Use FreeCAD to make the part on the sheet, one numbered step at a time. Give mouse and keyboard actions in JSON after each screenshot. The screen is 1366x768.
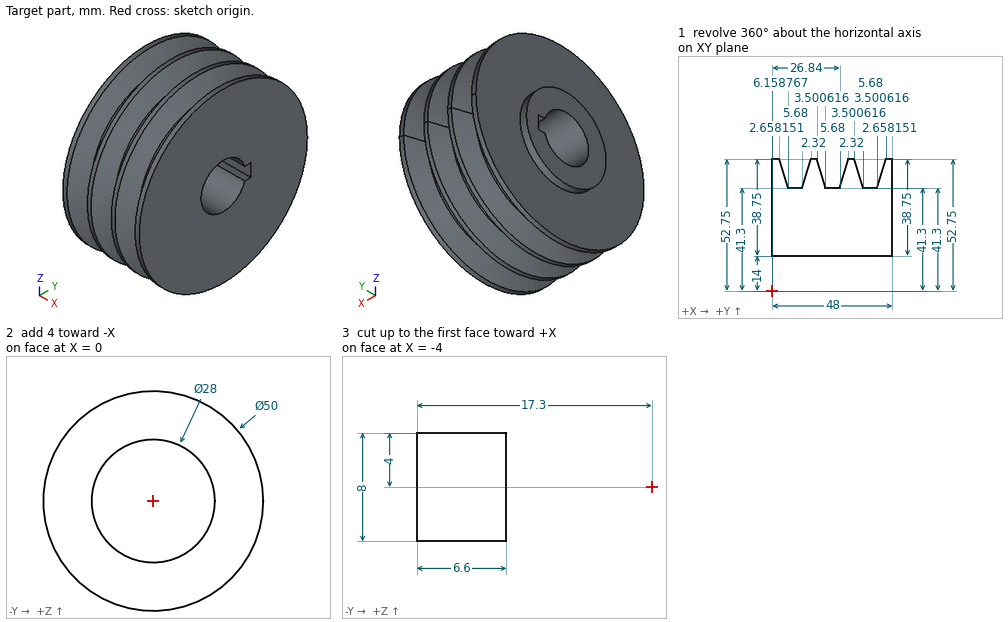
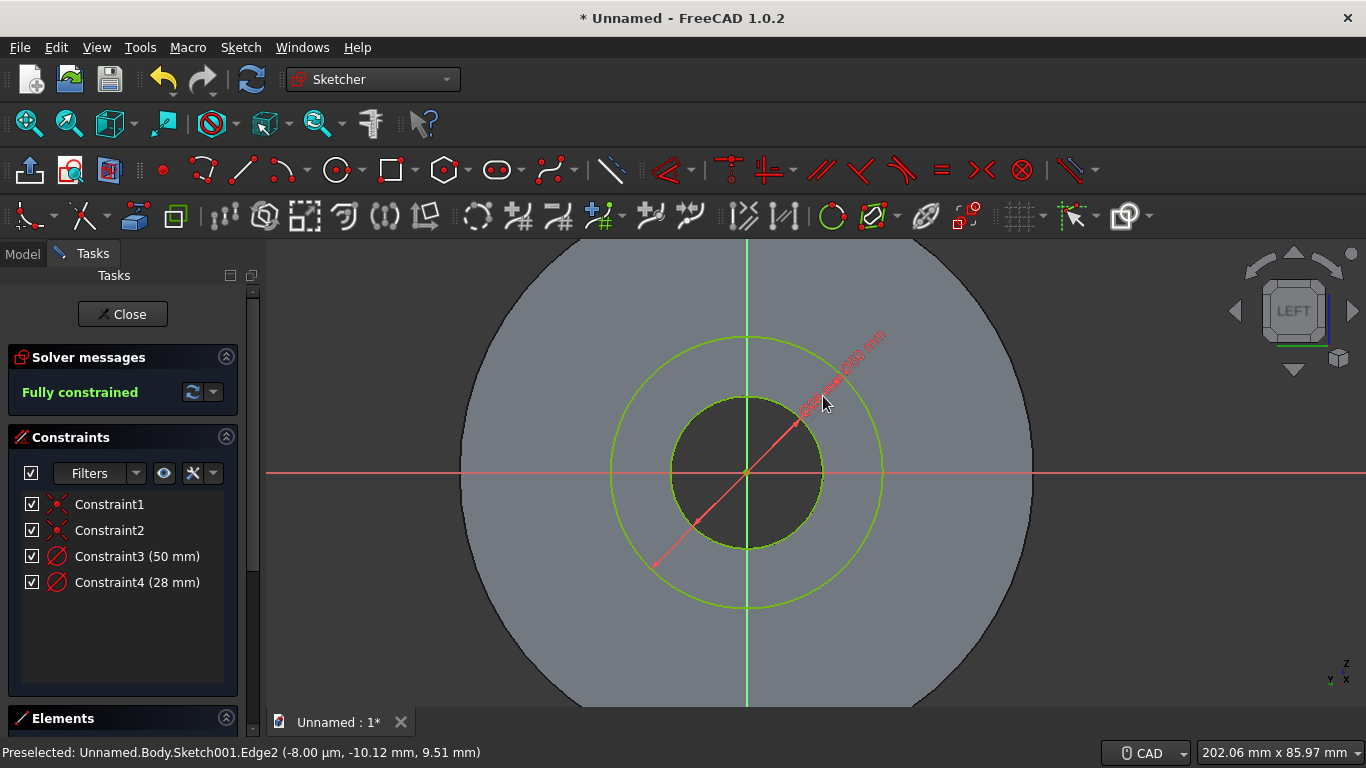
{"action": "left_click", "coordinate": [123, 314]}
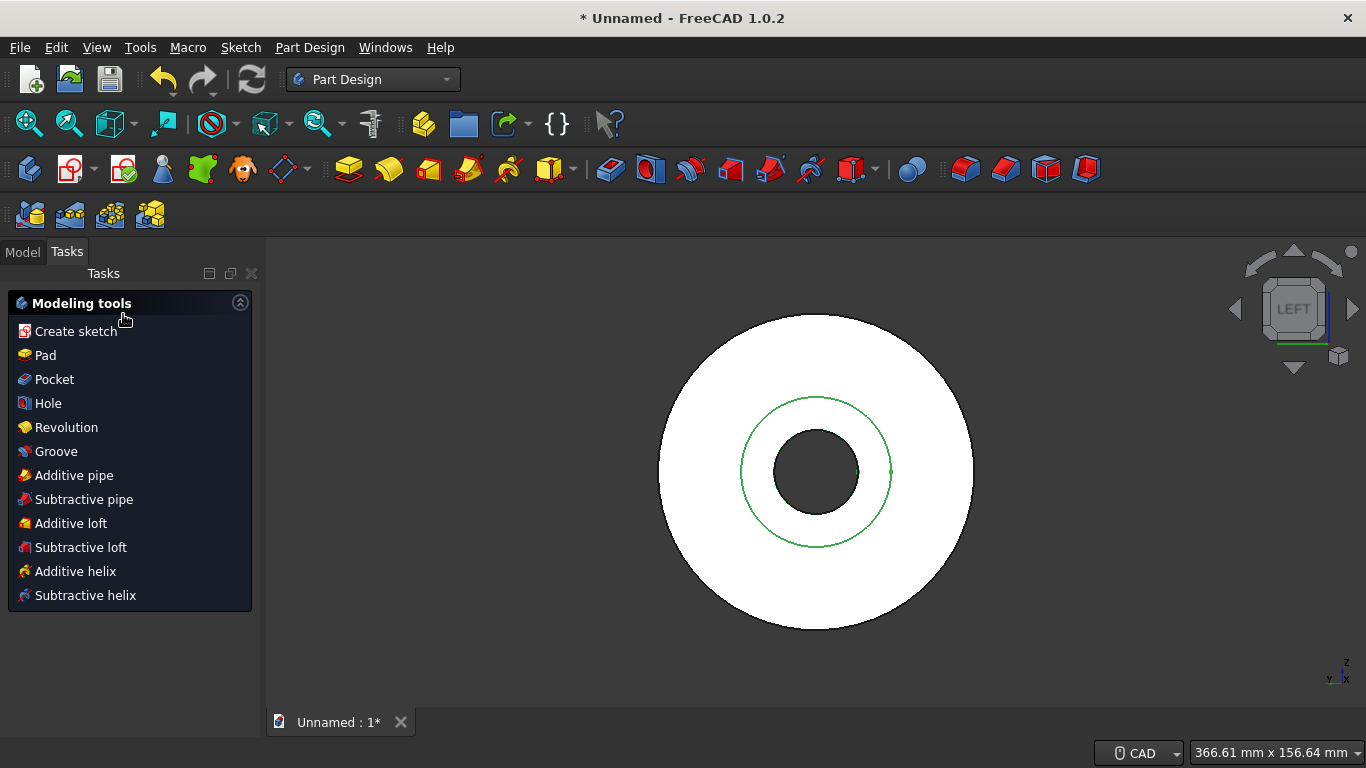
{"action": "left_click", "coordinate": [350, 170]}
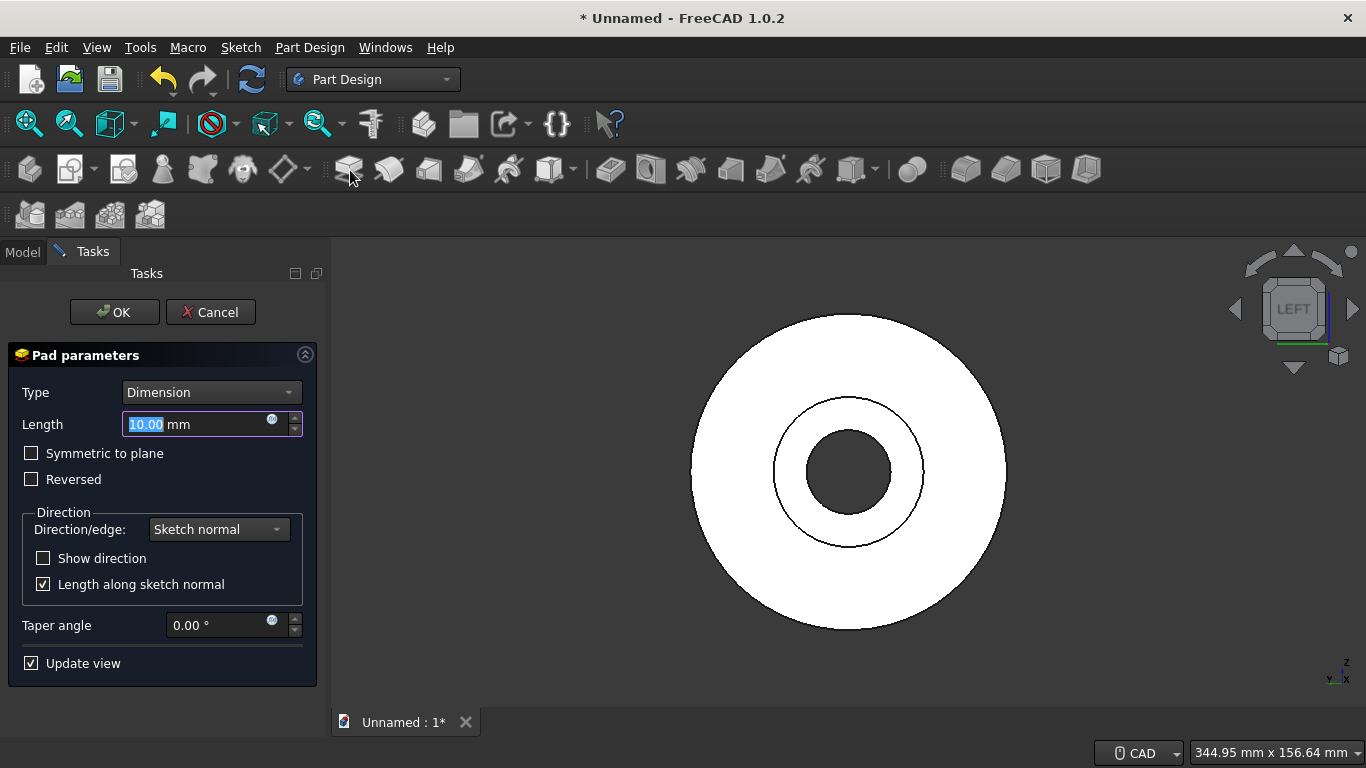
{"action": "type", "text": "4"}
{"action": "key", "text": "Tab"}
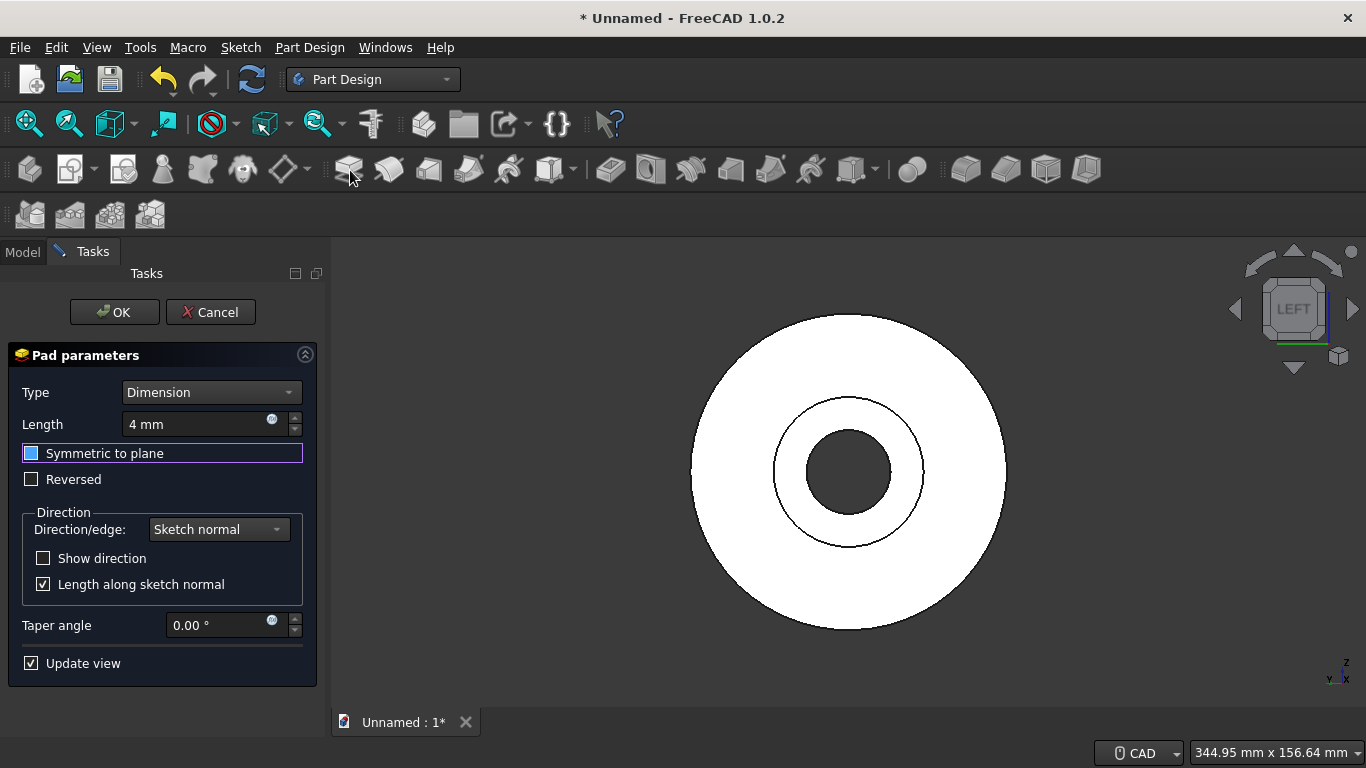
{"action": "left_click", "coordinate": [115, 312]}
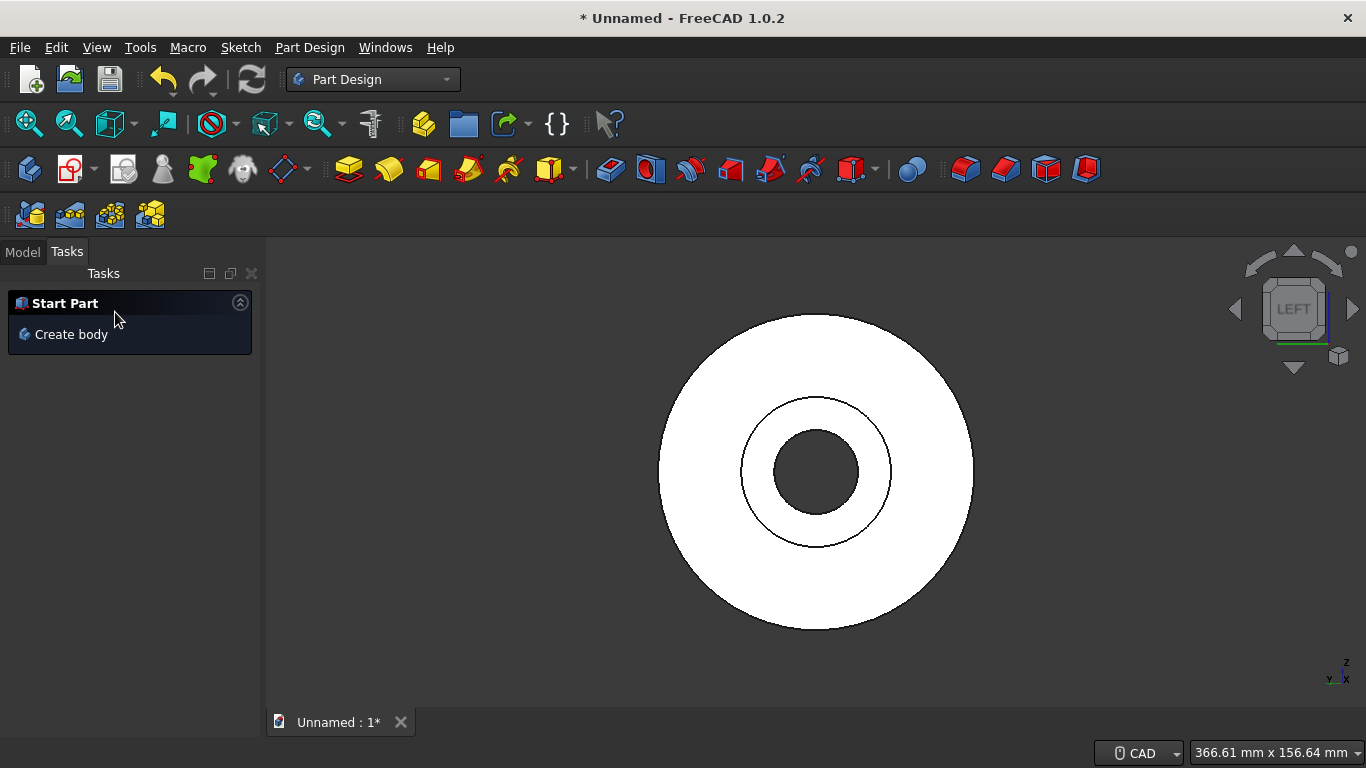
{"action": "left_click", "coordinate": [859, 514]}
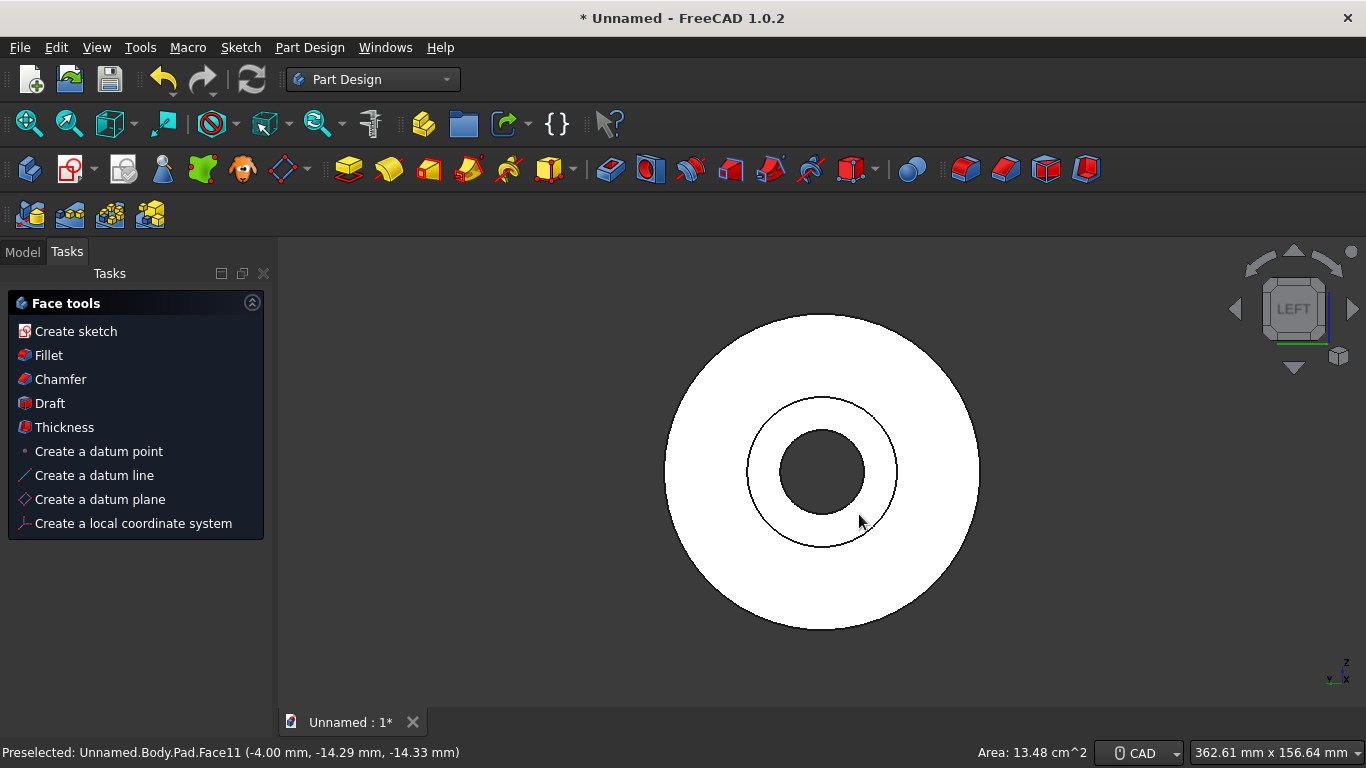
{"action": "left_click", "coordinate": [70, 170]}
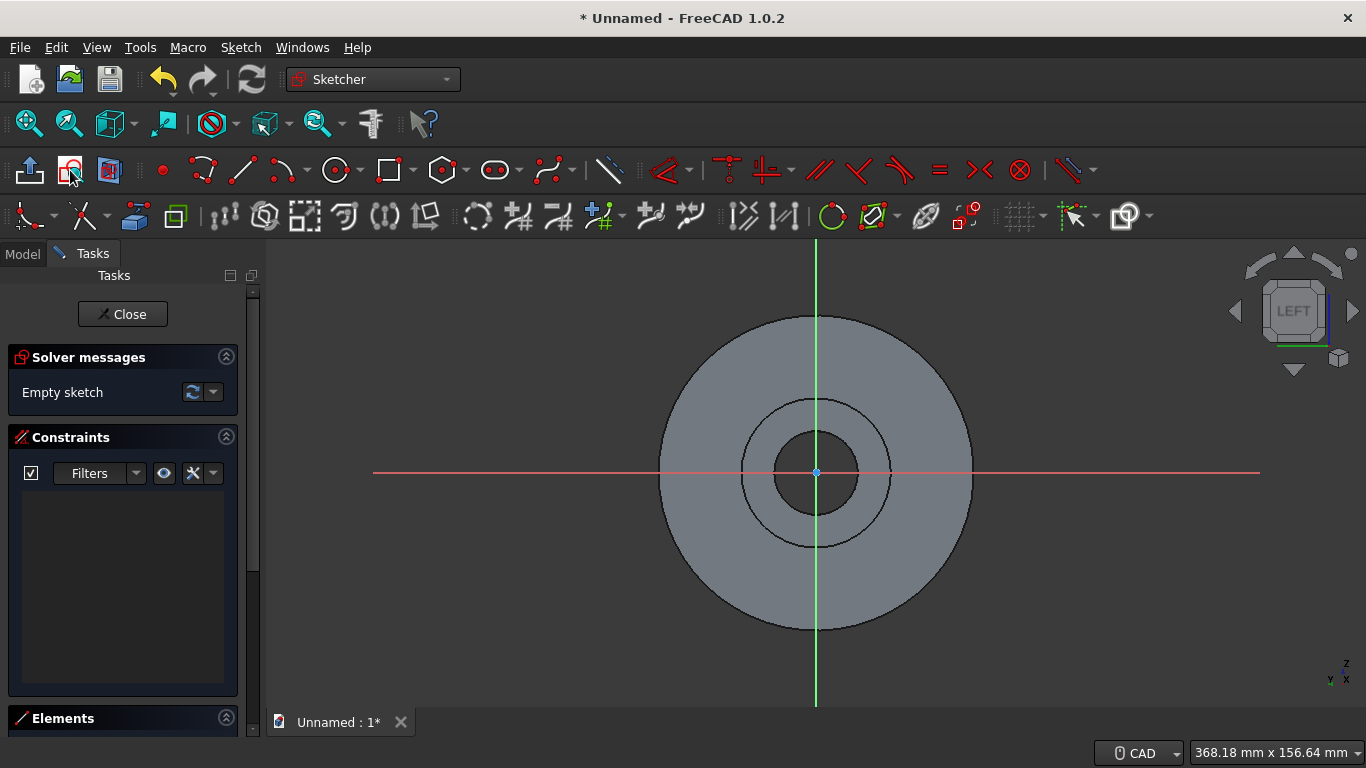
{"action": "scroll", "coordinate": [795, 473], "scroll_direction": "up", "scroll_amount": 12}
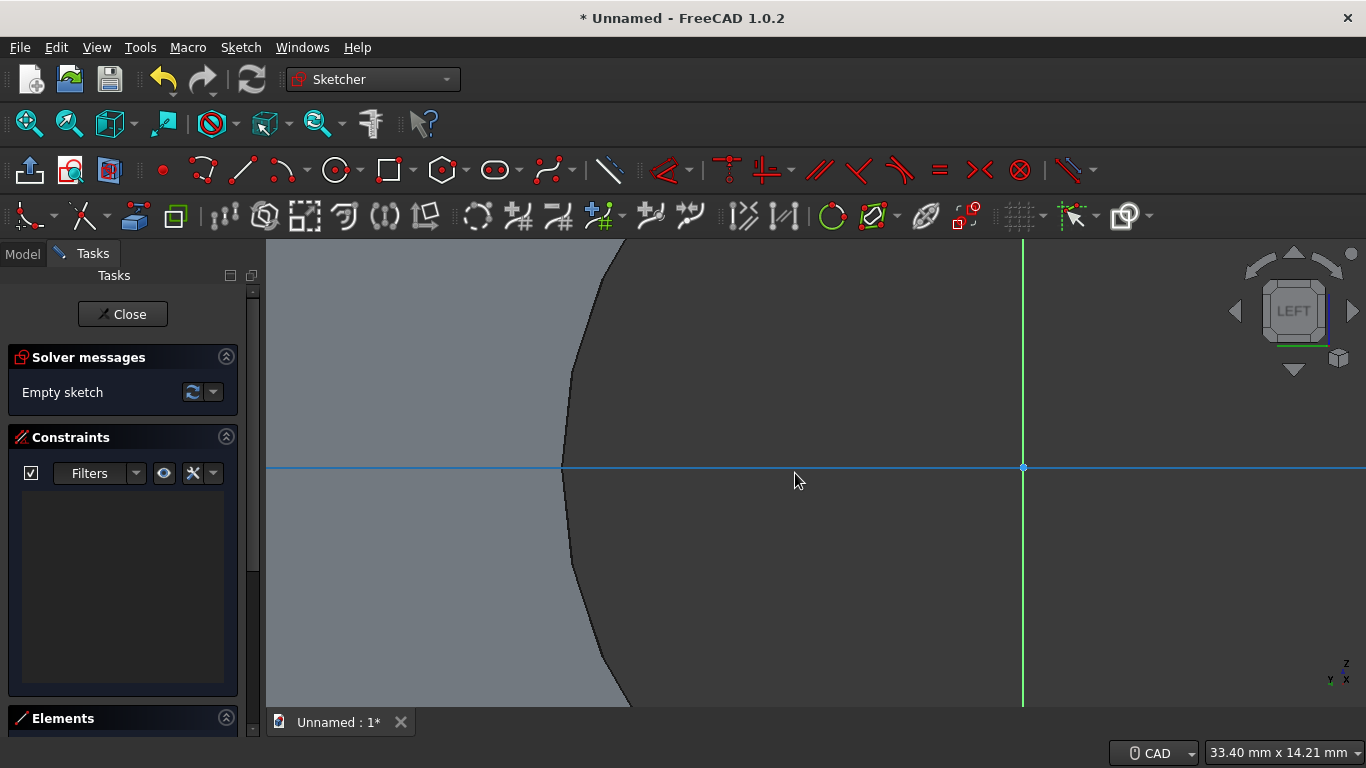
{"action": "left_click", "coordinate": [390, 170]}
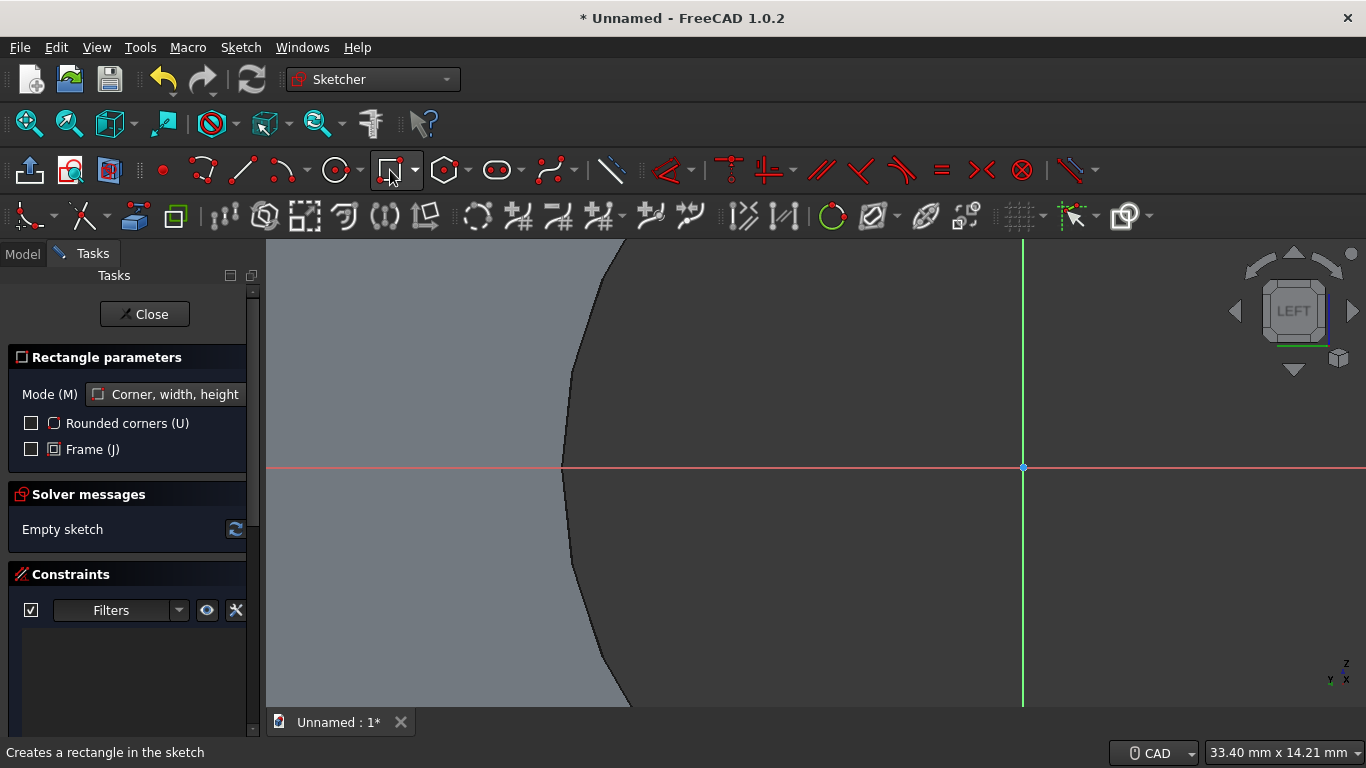
{"action": "left_click", "coordinate": [453, 336]}
{"action": "left_click", "coordinate": [671, 600]}
{"action": "key", "text": "Escape"}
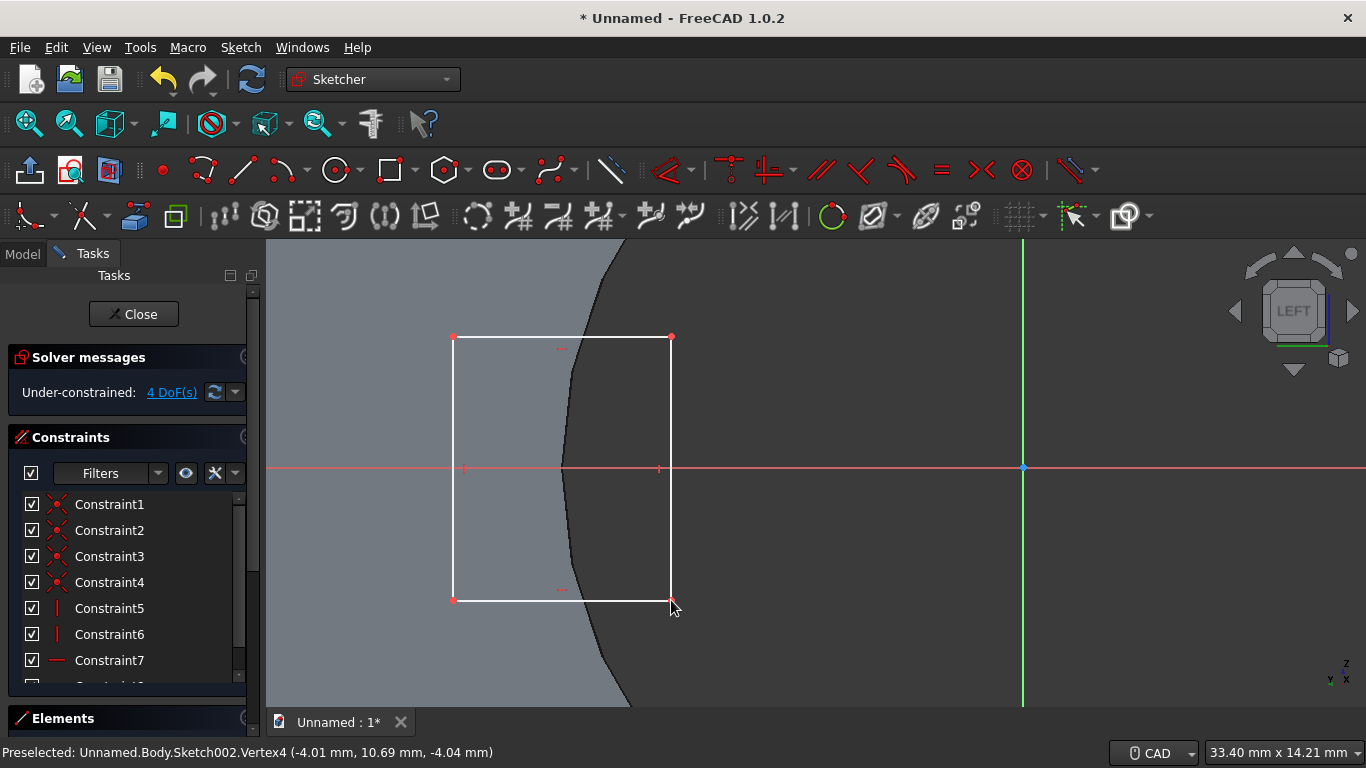
{"action": "left_click", "coordinate": [666, 170]}